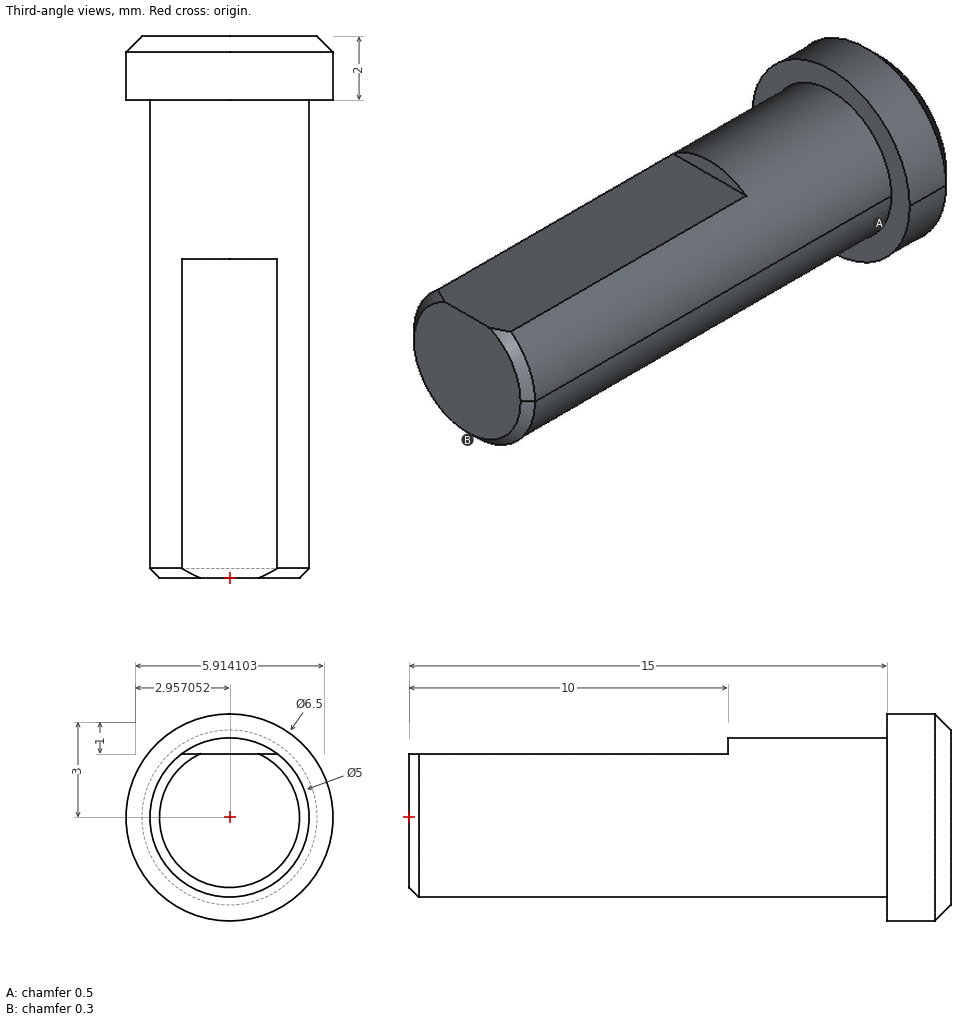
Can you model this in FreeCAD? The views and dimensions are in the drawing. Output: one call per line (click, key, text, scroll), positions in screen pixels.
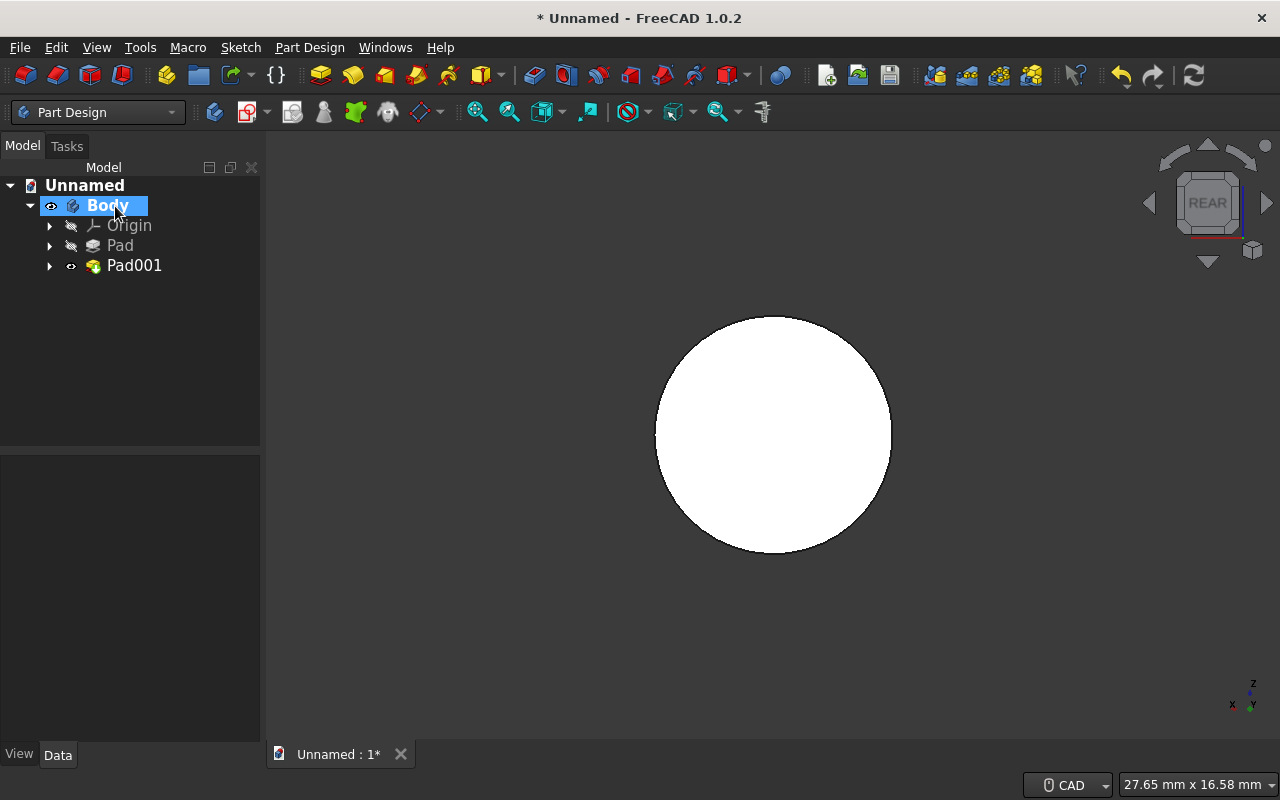
click(478, 112)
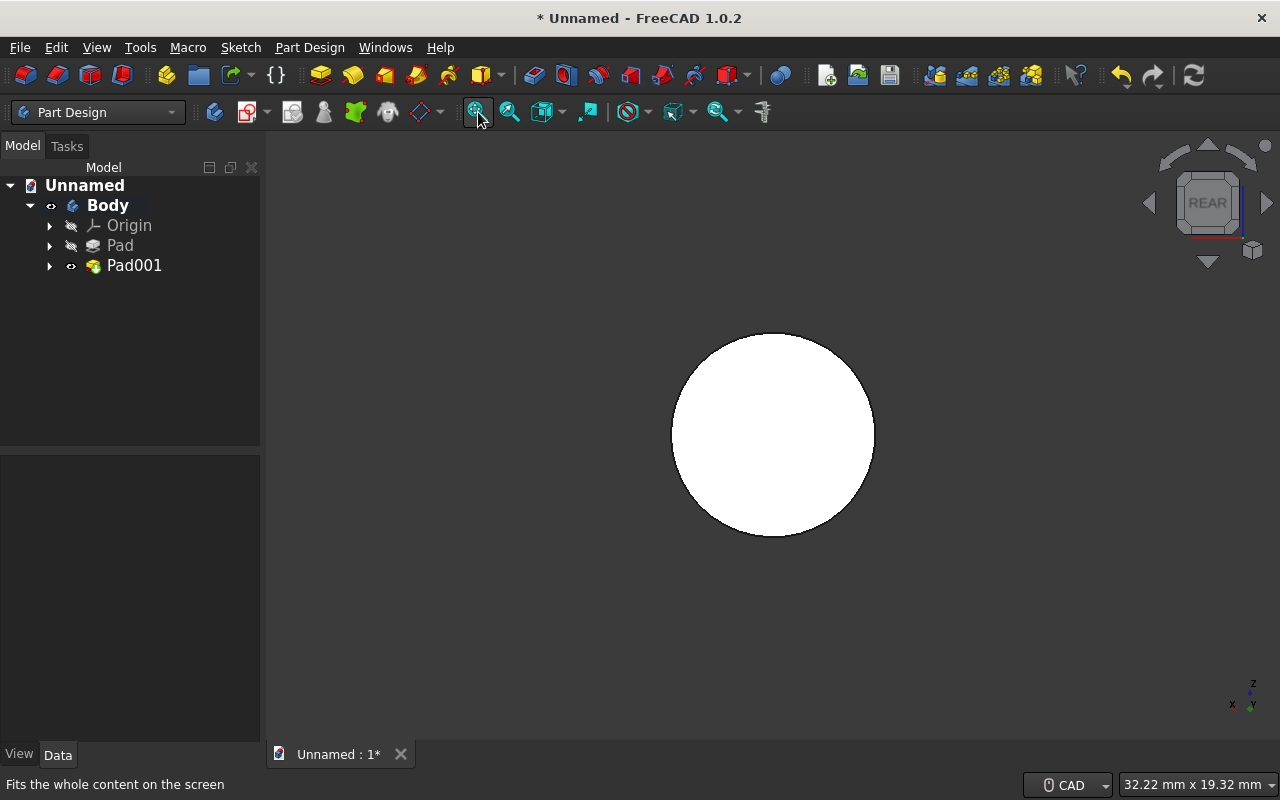
click(875, 434)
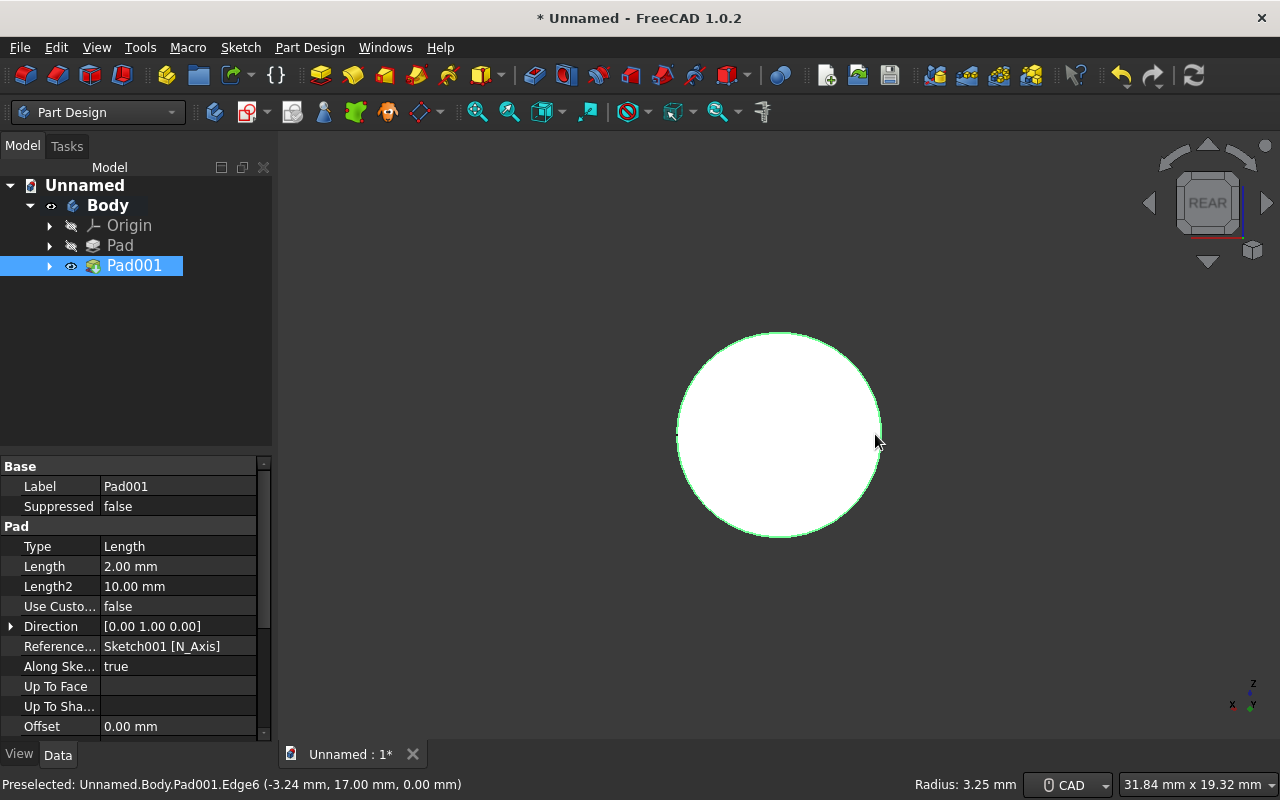
click(58, 76)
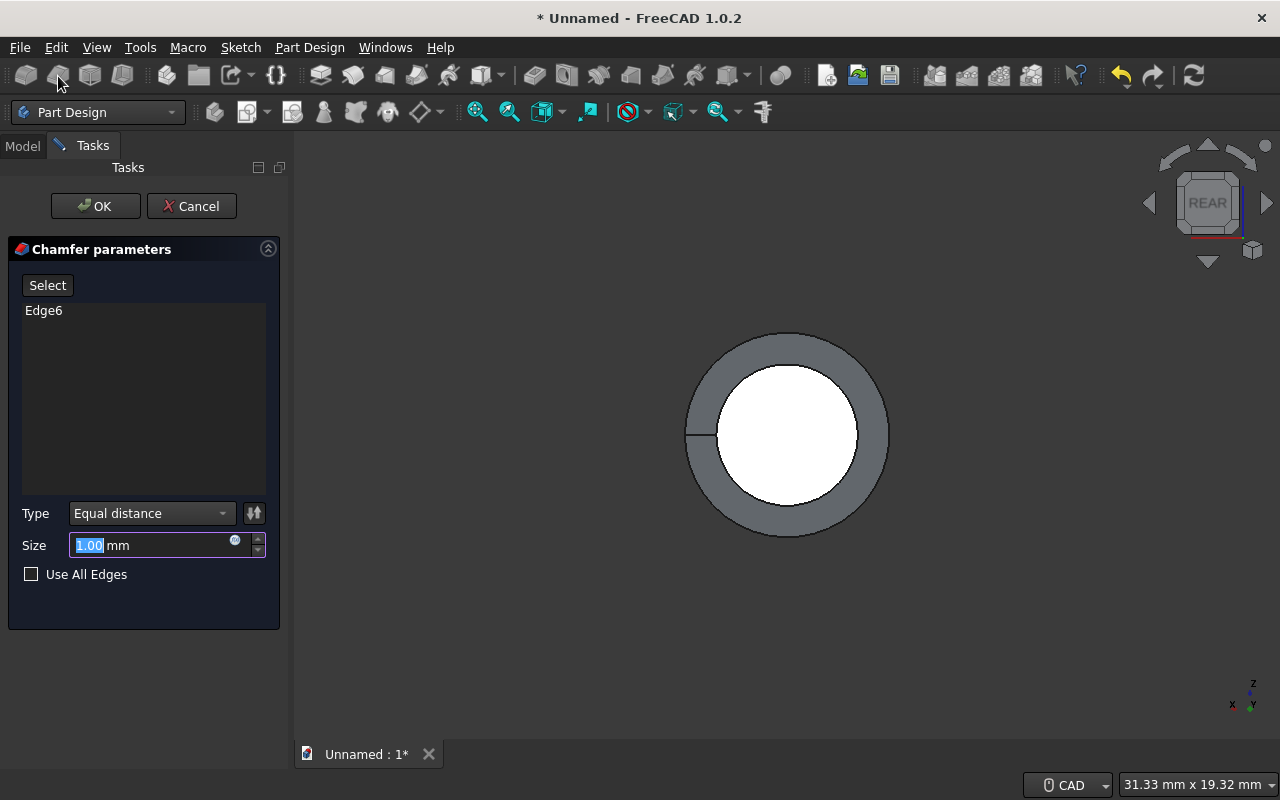
text(0.5)
key(Tab)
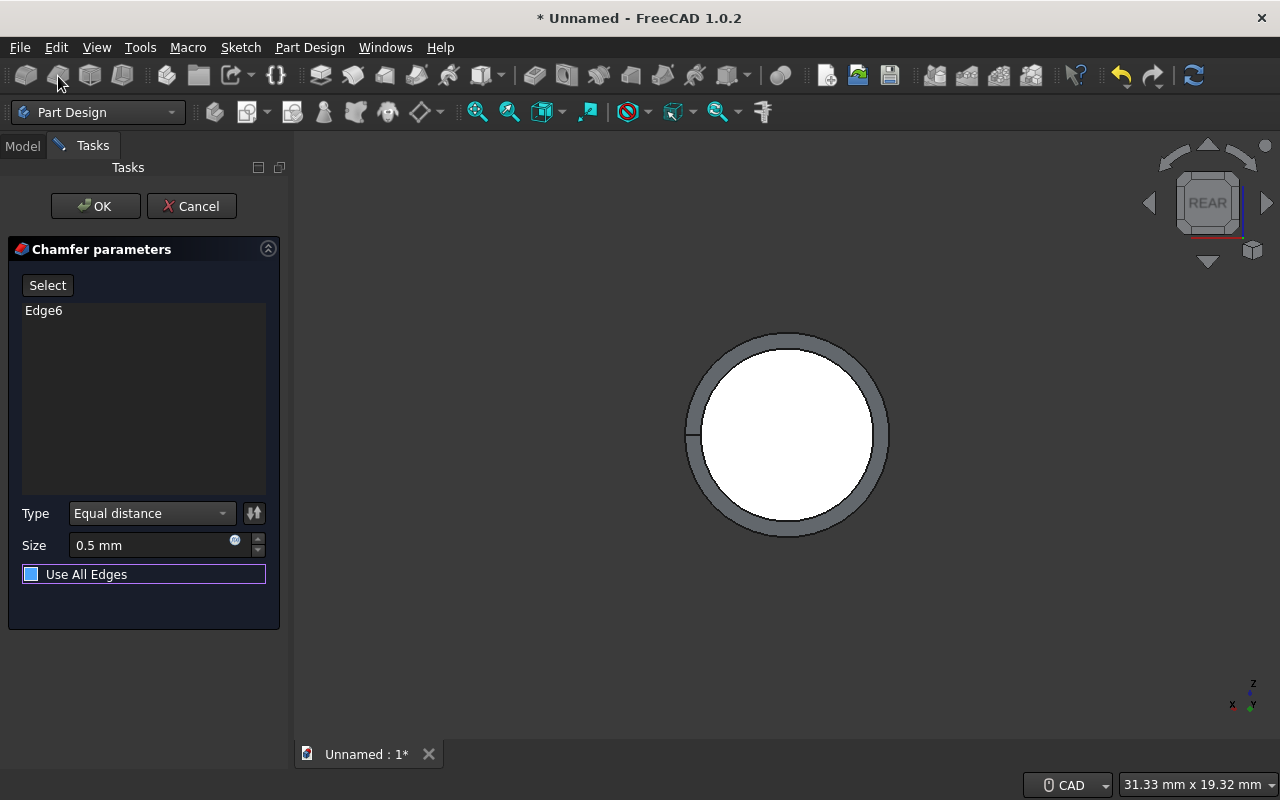
click(96, 206)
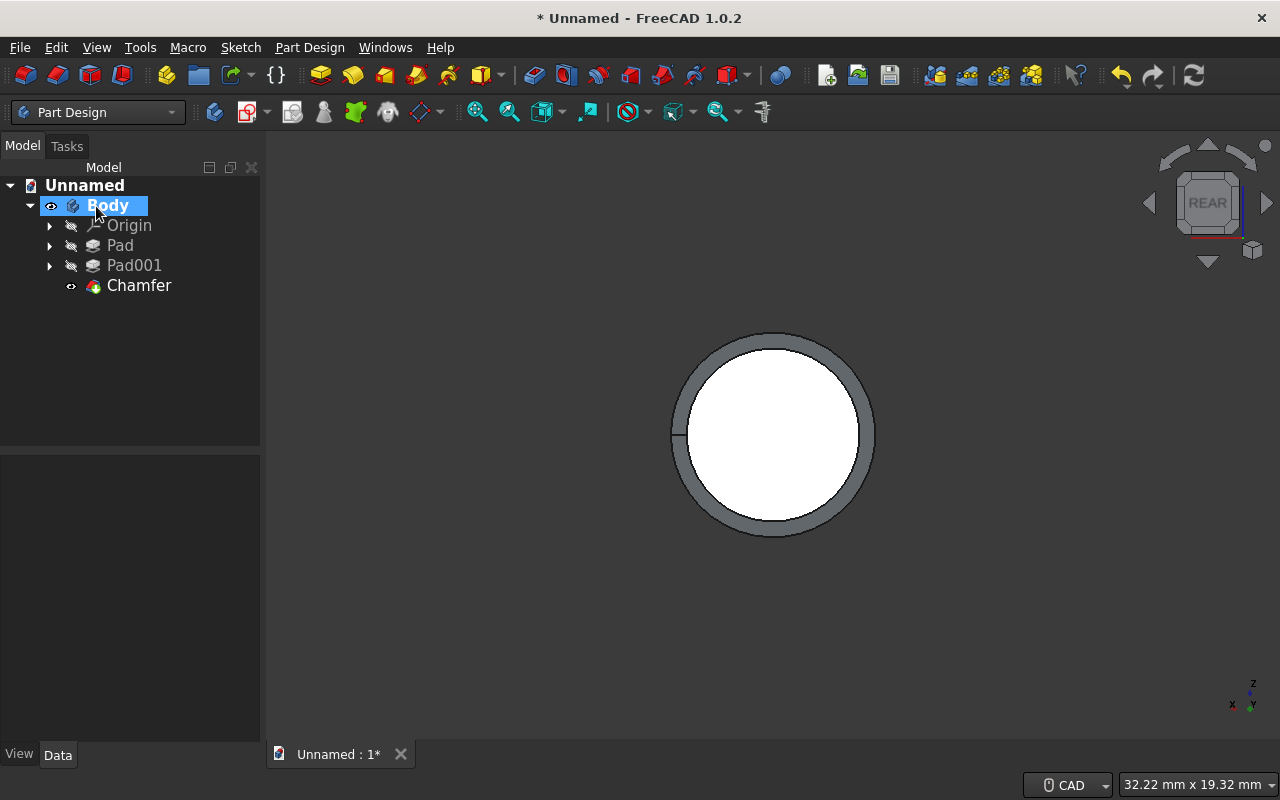
click(478, 112)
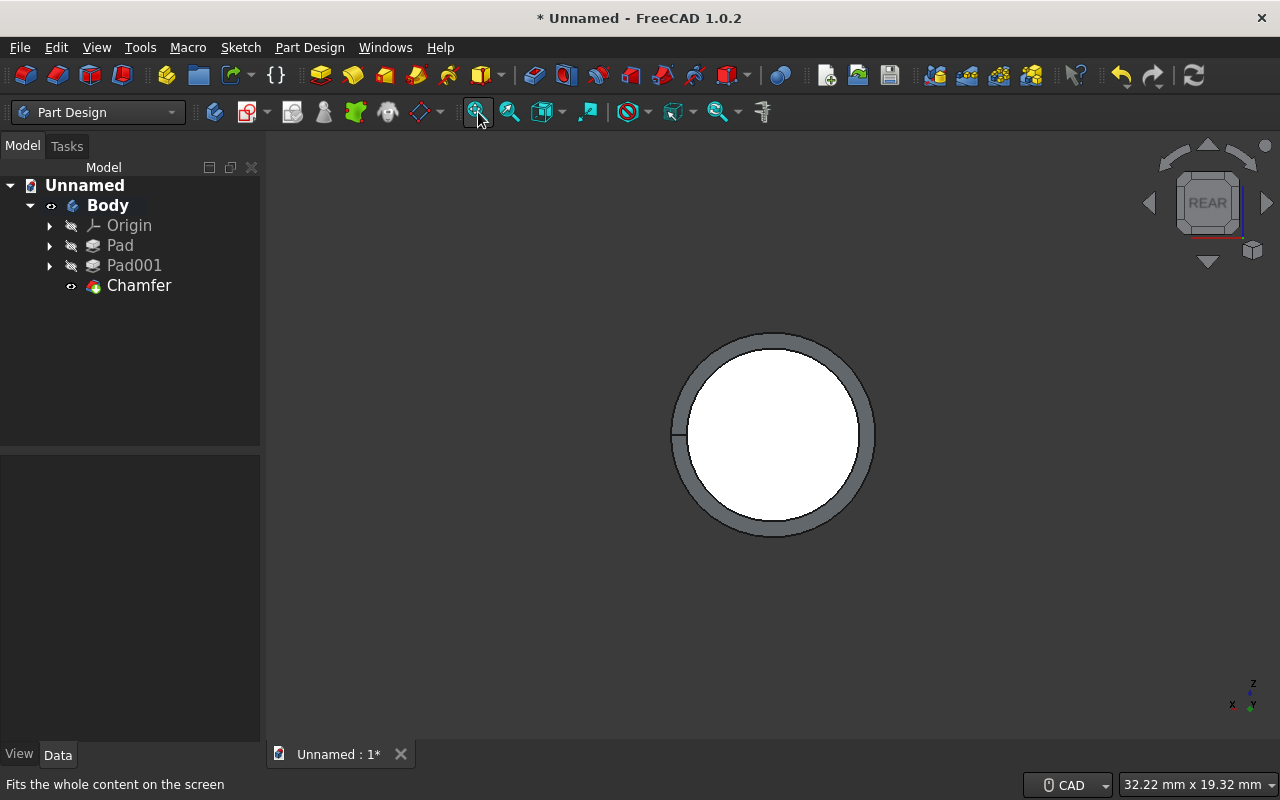
key(0)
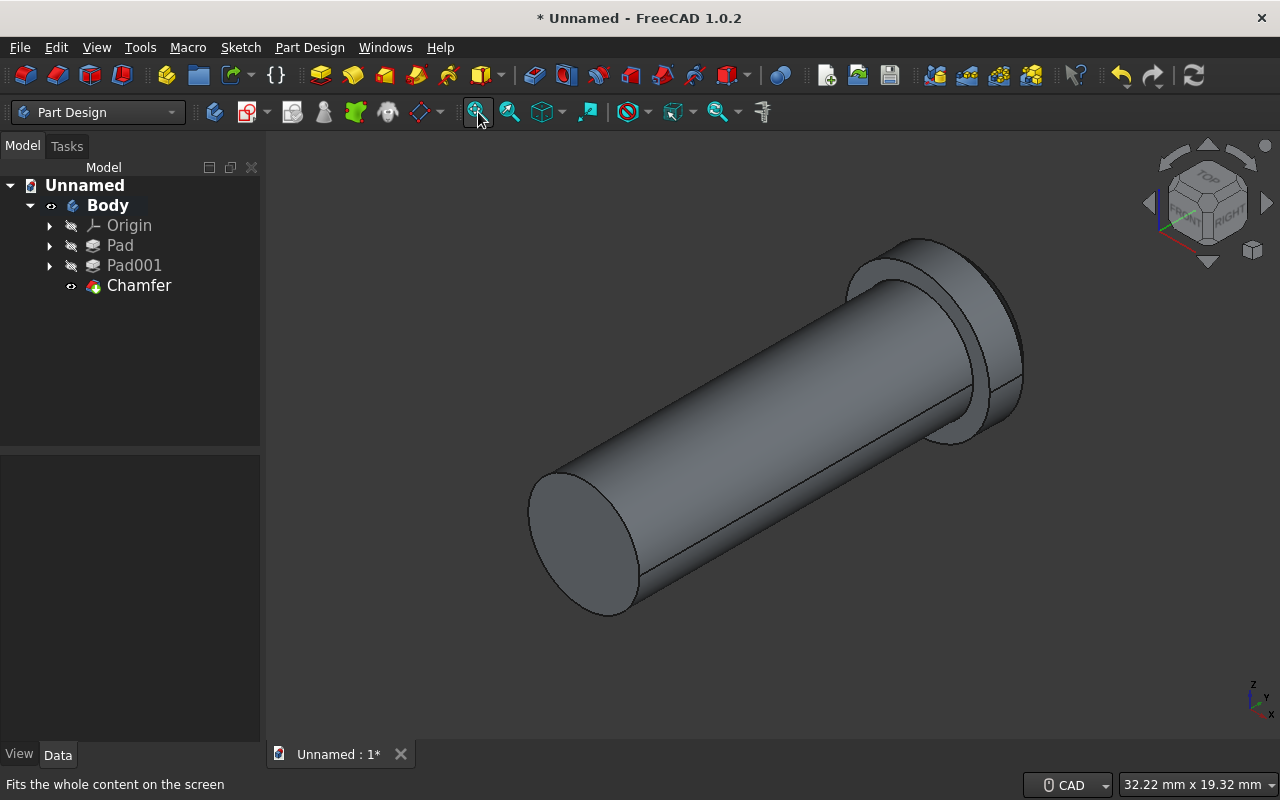
click(539, 479)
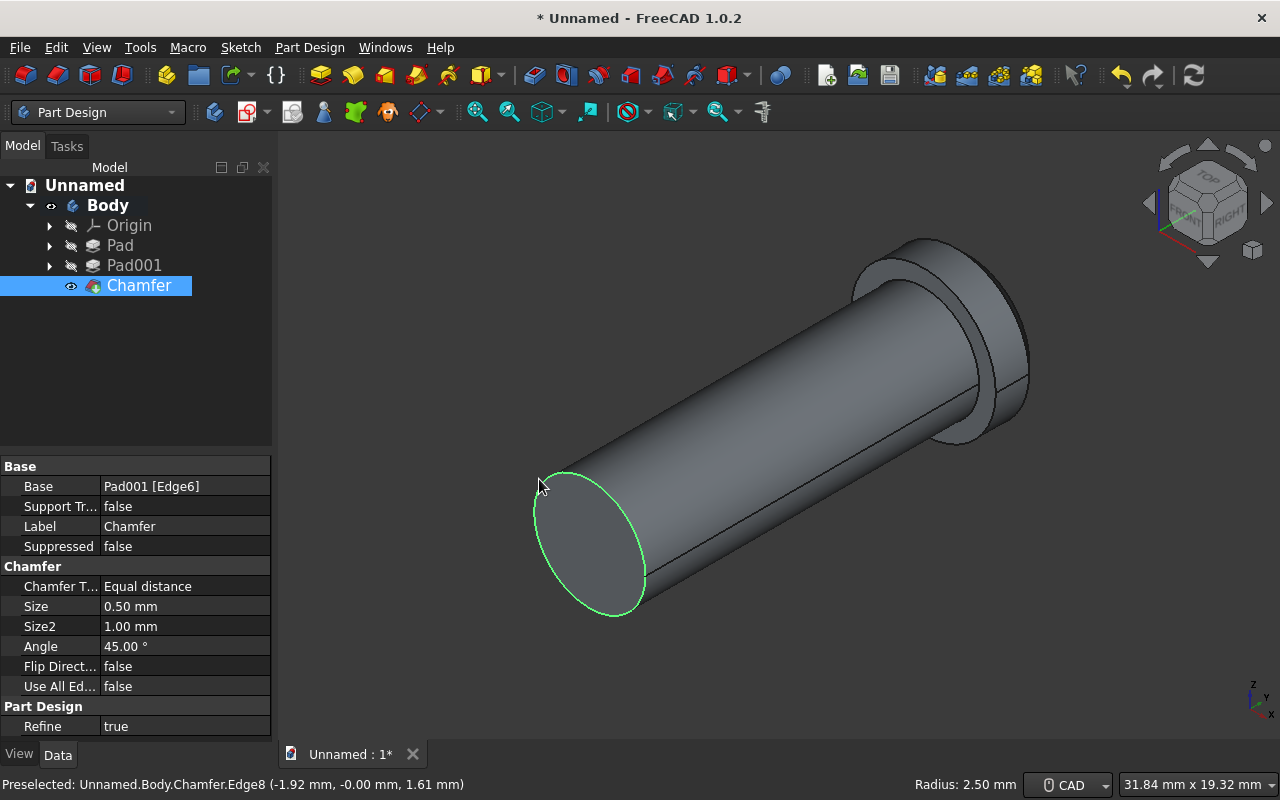
click(58, 76)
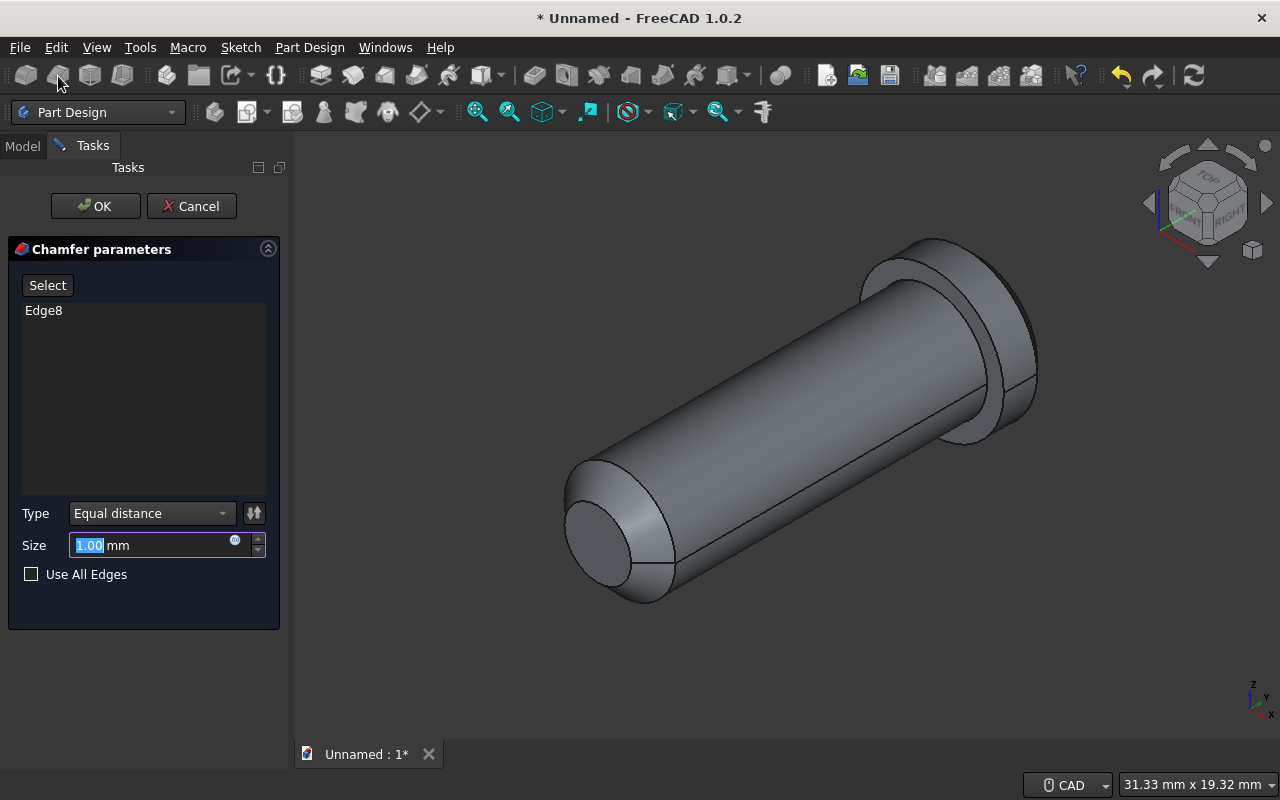
text(0.3)
key(Tab)